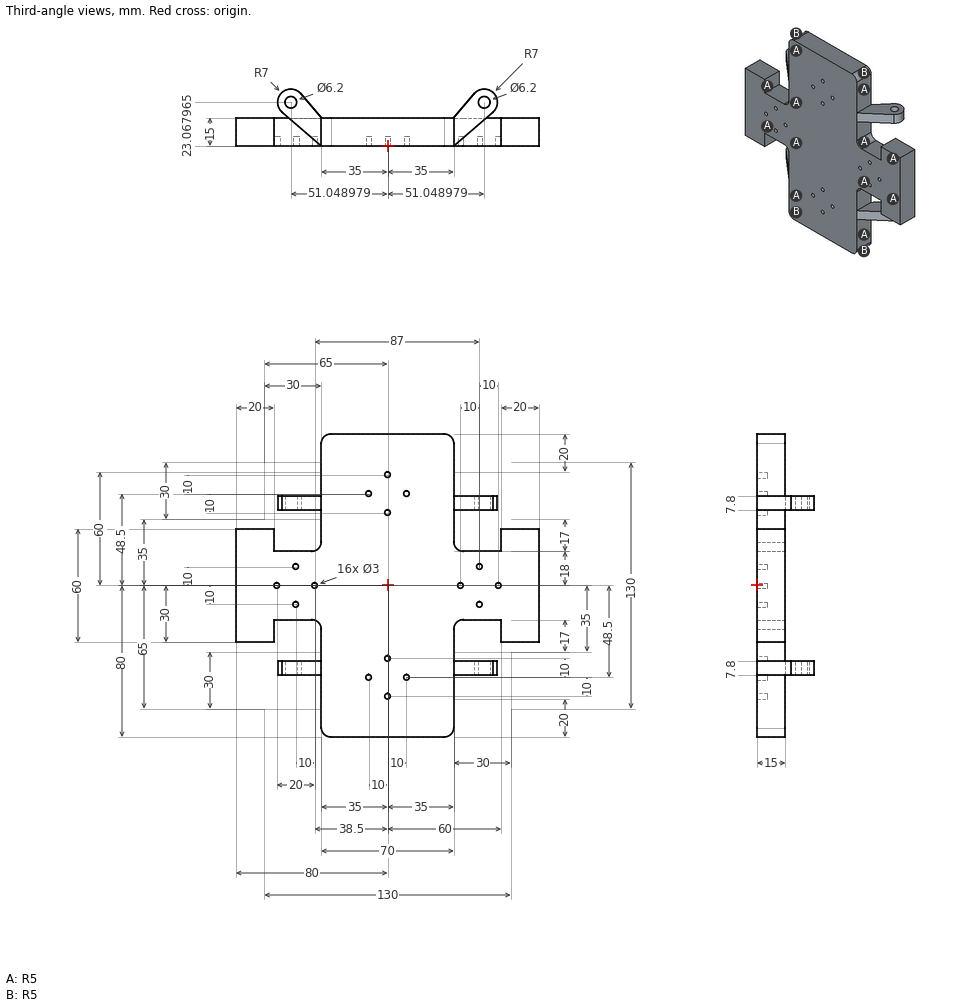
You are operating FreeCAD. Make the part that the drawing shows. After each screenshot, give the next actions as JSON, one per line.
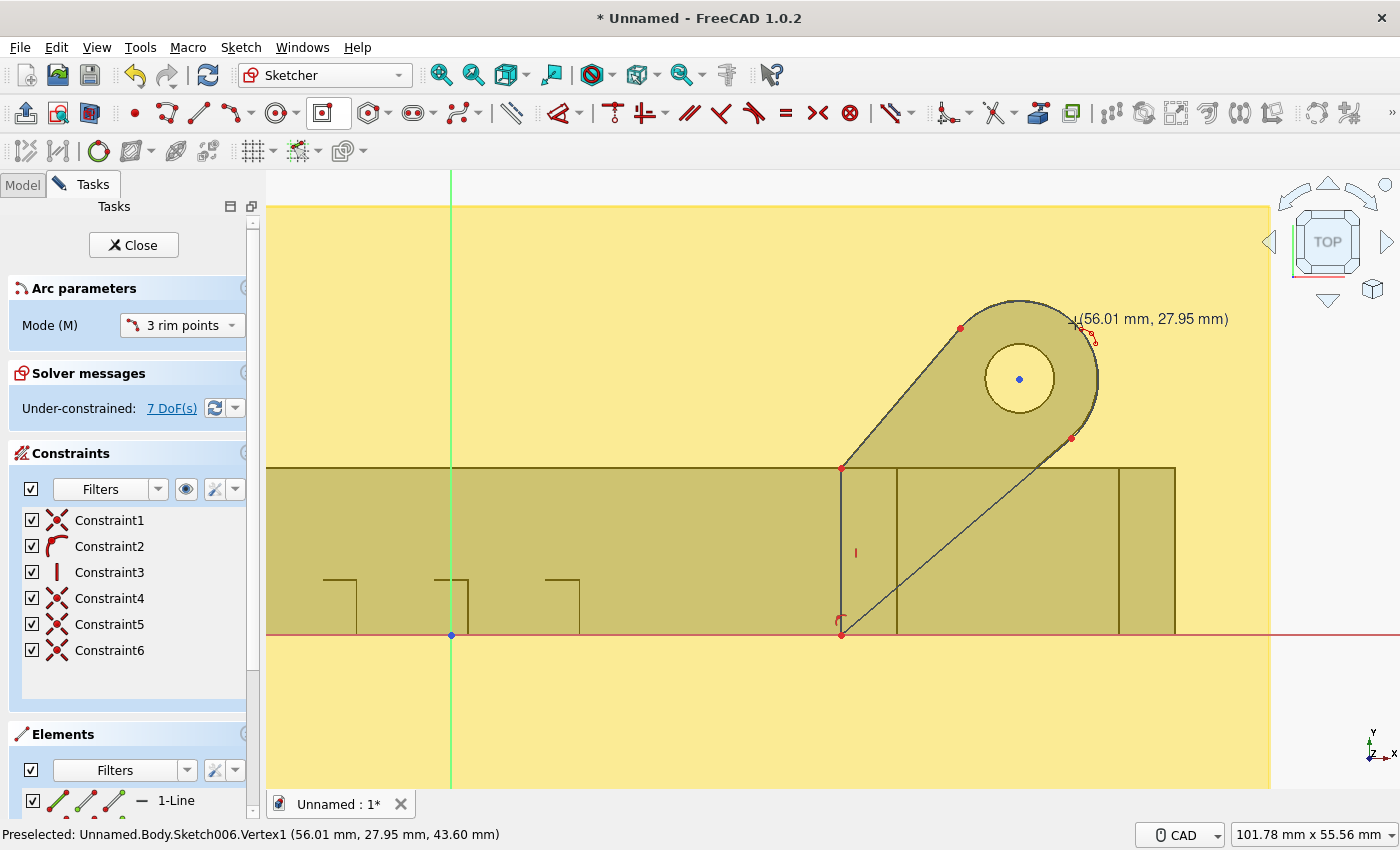
{"action": "left_click", "coordinate": [276, 114]}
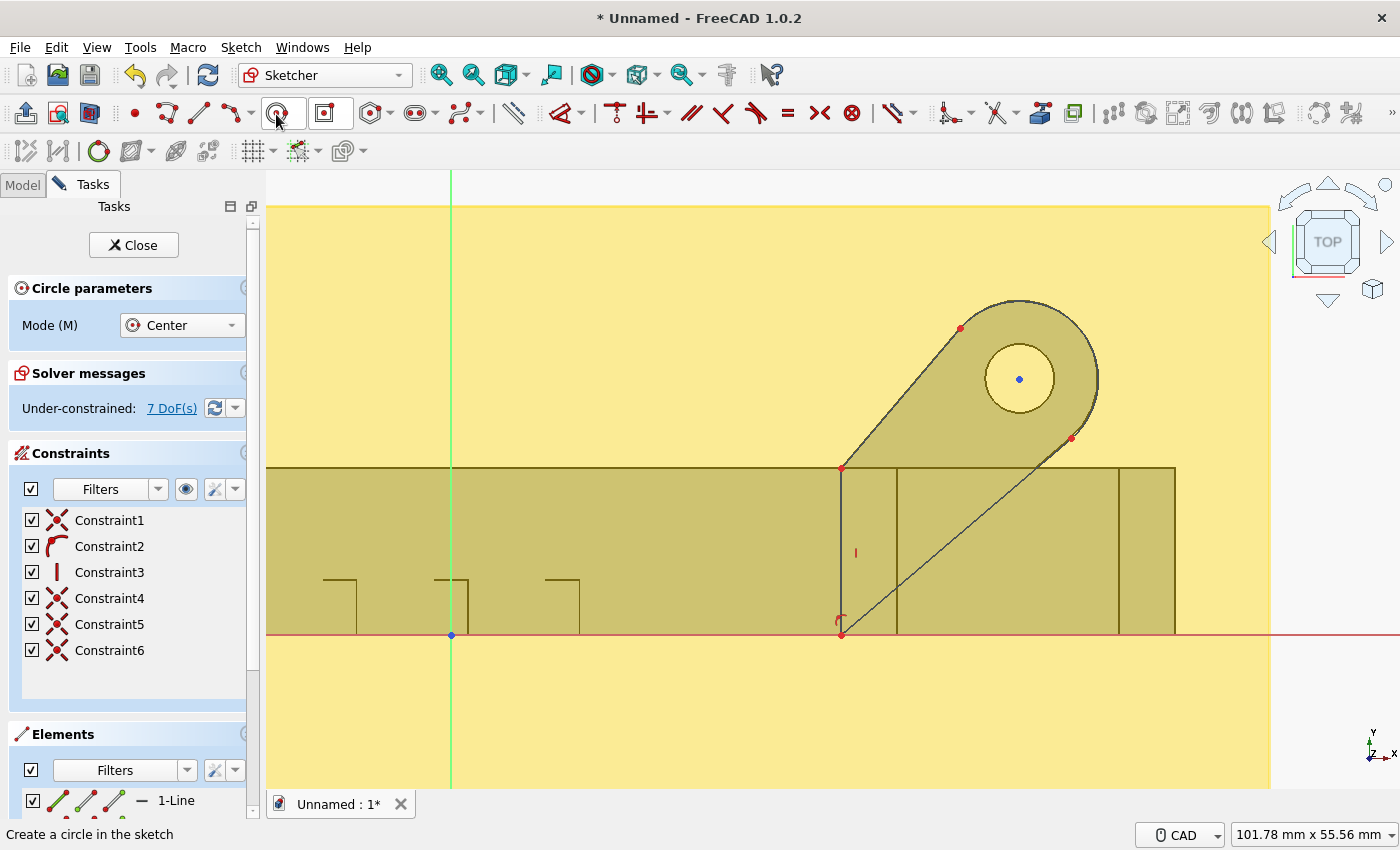
{"action": "left_click", "coordinate": [1020, 378]}
{"action": "mouse_move", "coordinate": [1044, 354]}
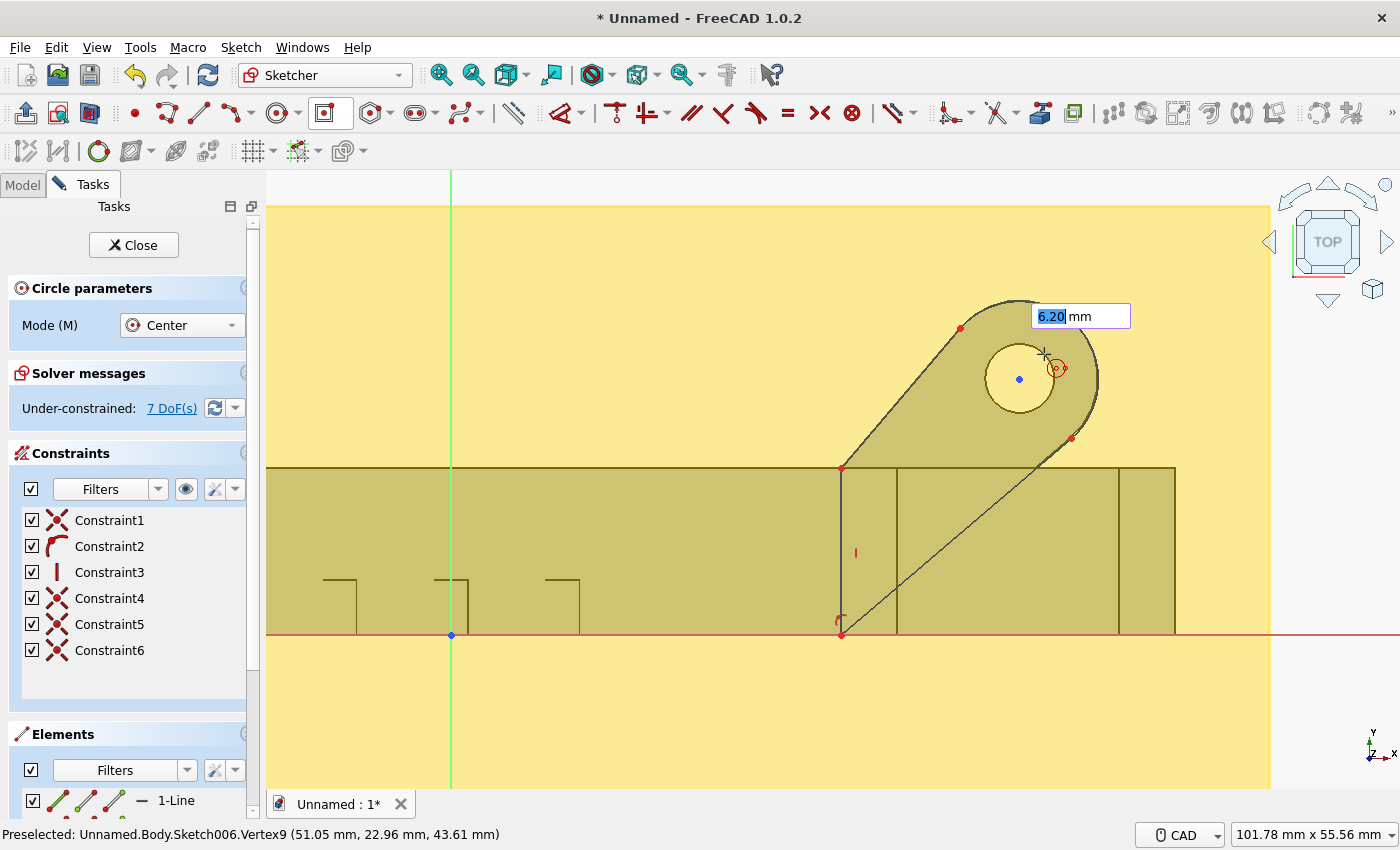
{"action": "type", "text": "6.2"}
{"action": "key", "text": "Return"}
{"action": "key", "text": "Escape"}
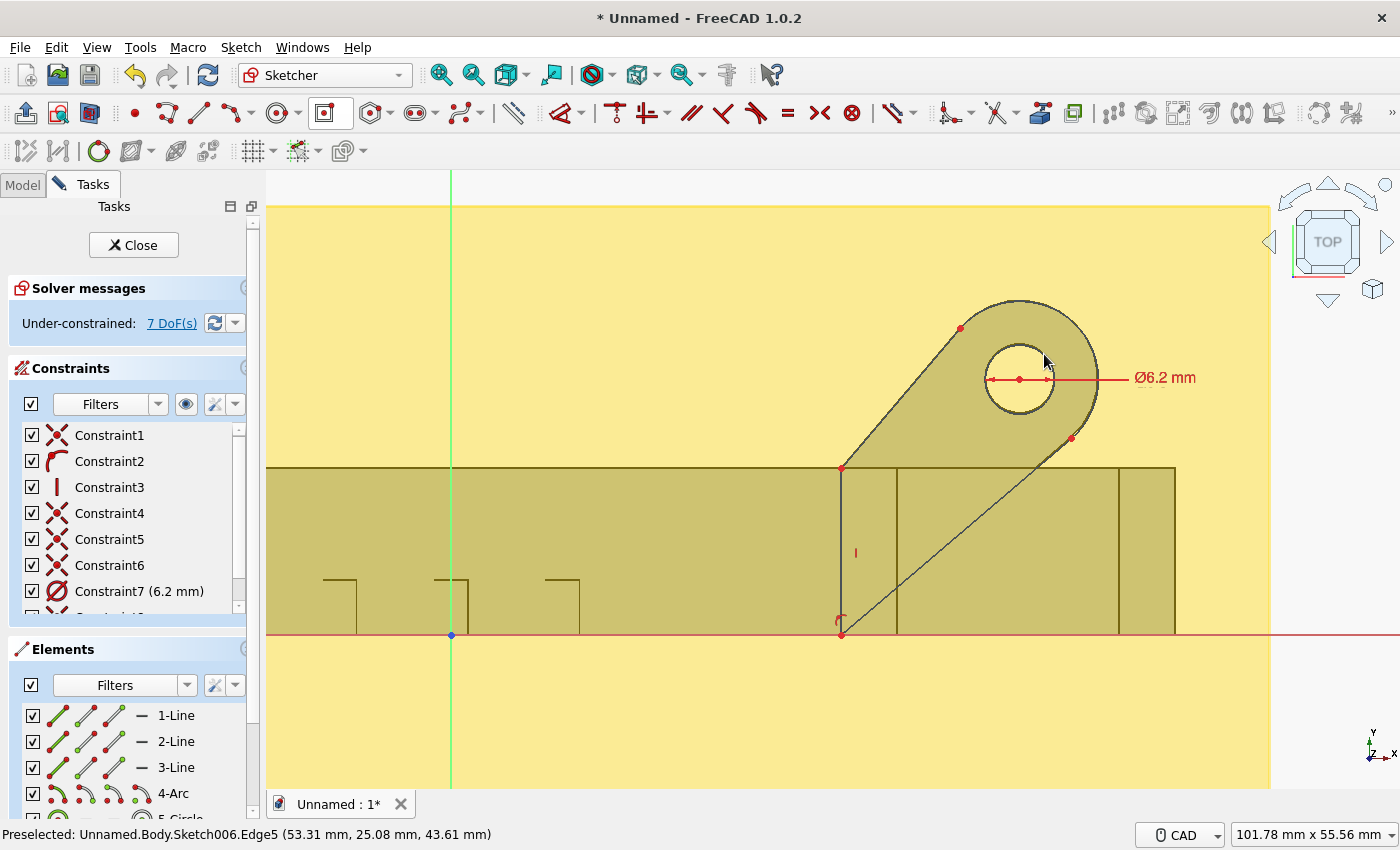
{"action": "left_click", "coordinate": [924, 371]}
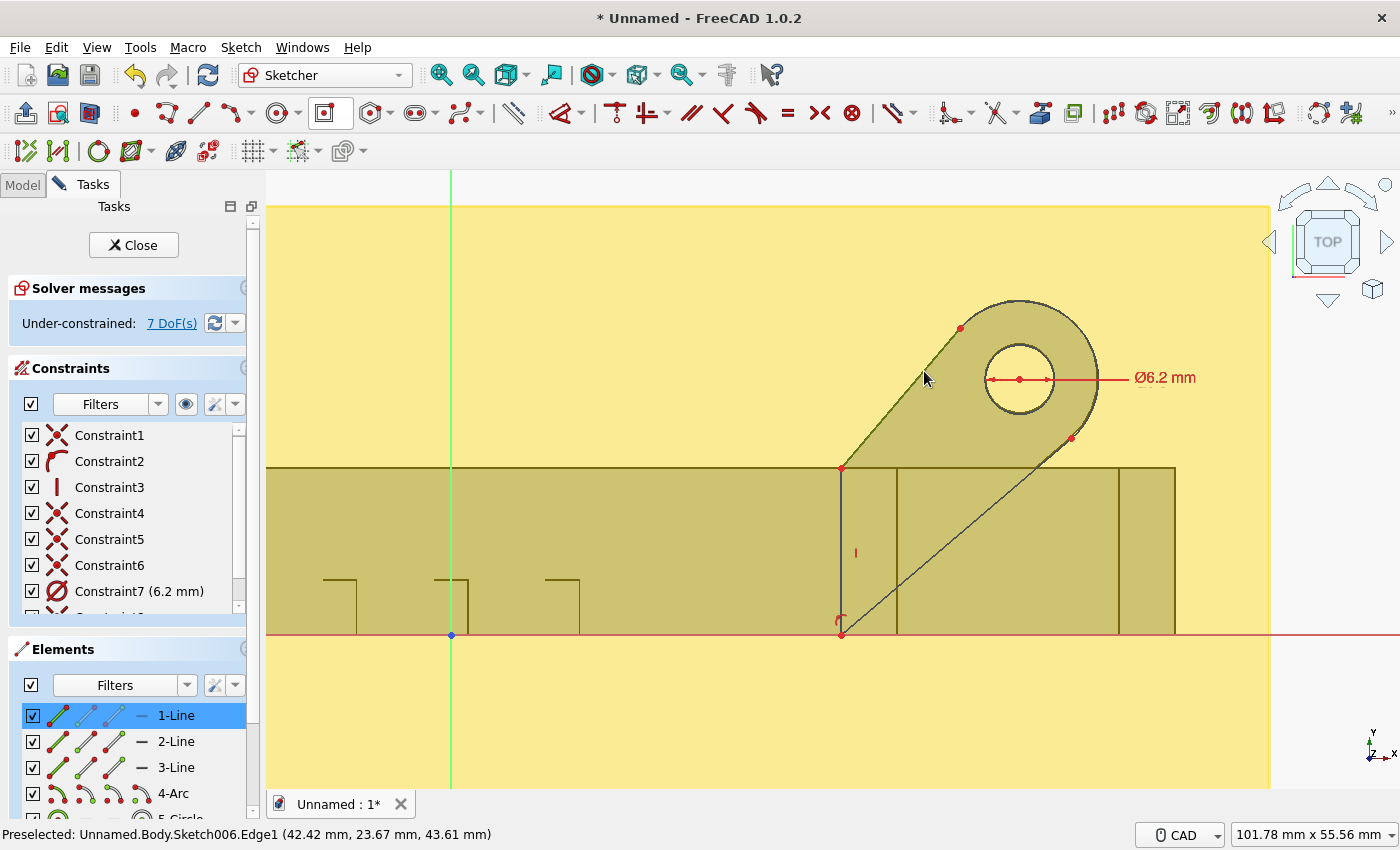
{"action": "left_click", "coordinate": [1098, 369]}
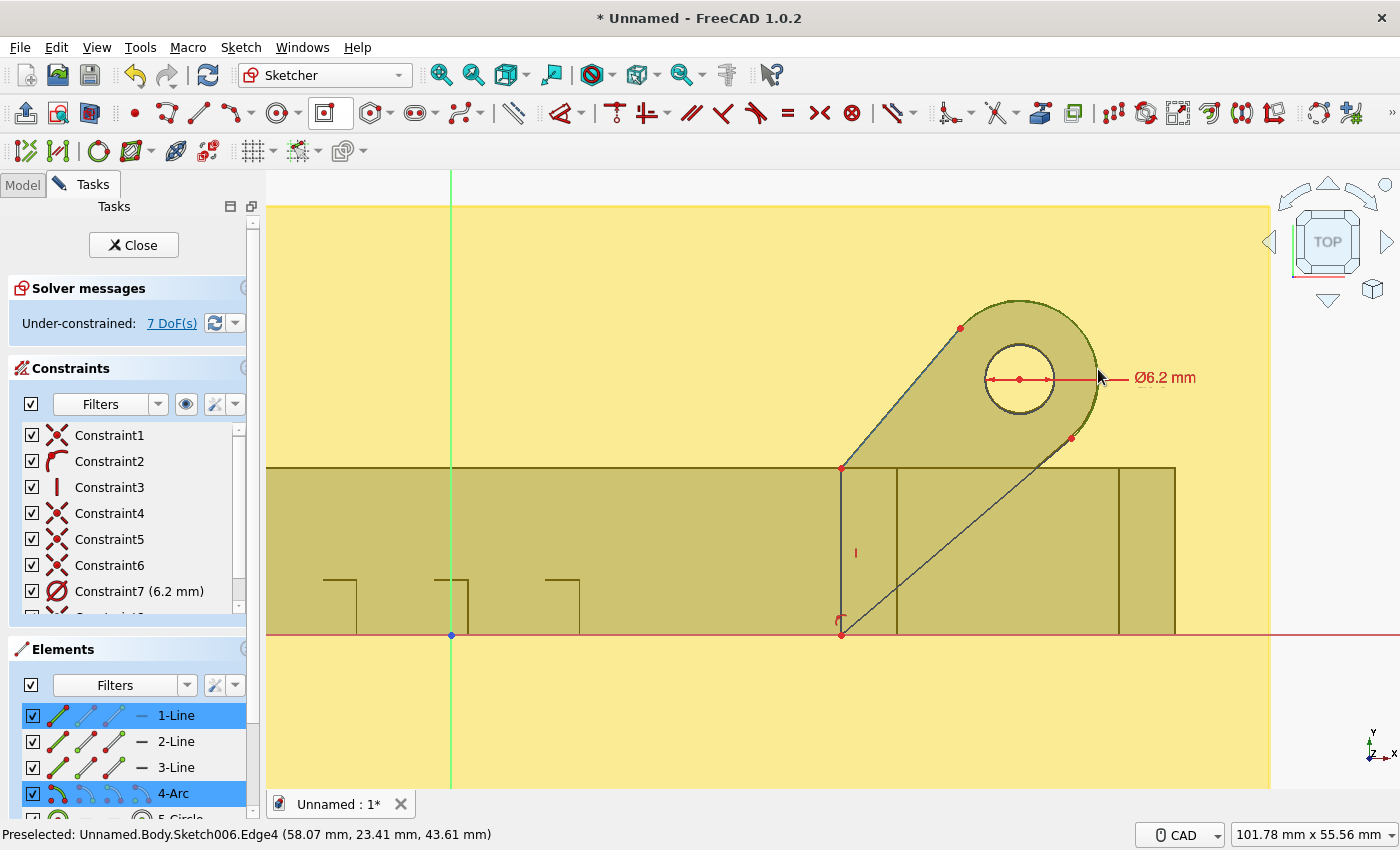
{"action": "key", "text": "t"}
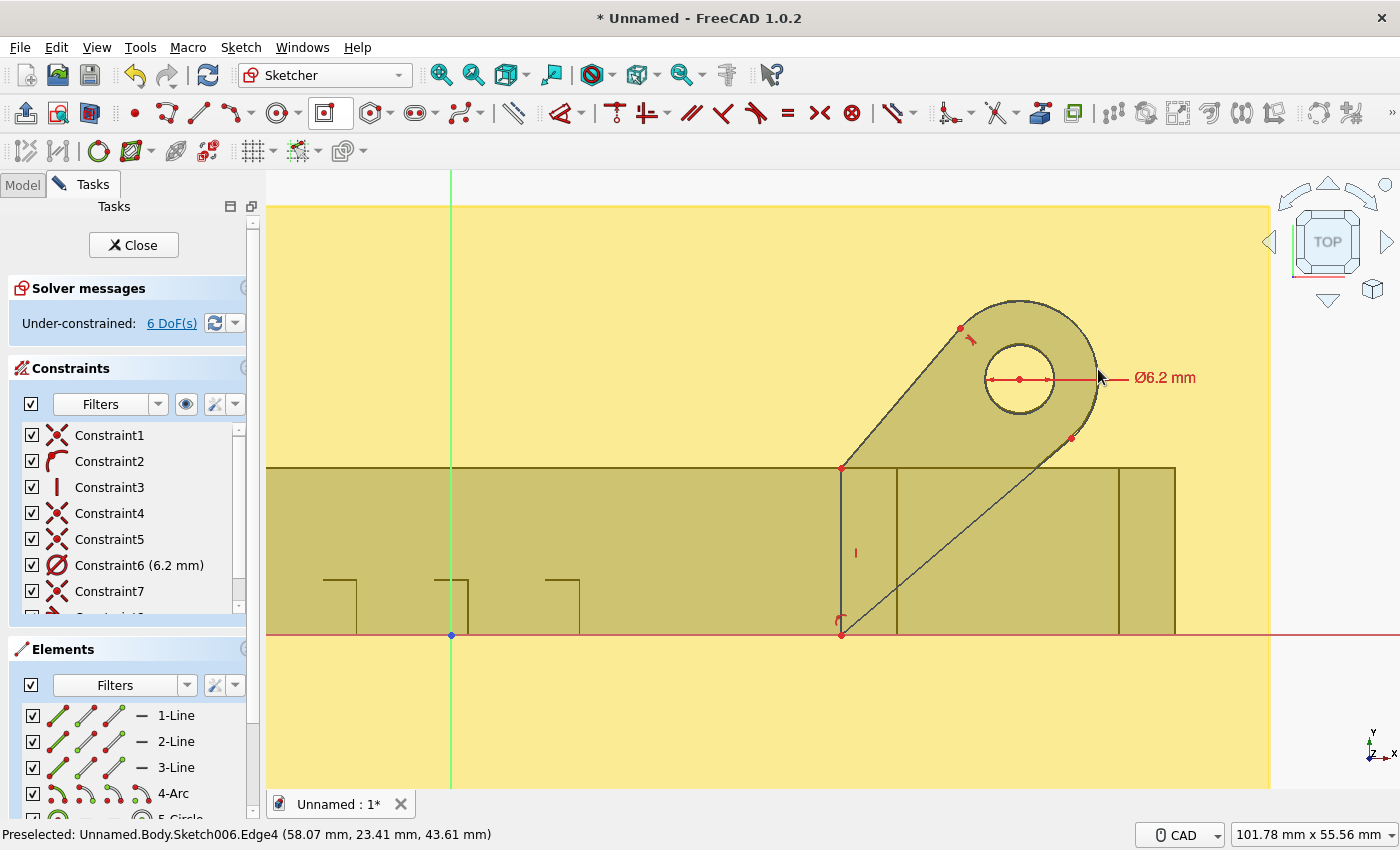
{"action": "left_click", "coordinate": [910, 577]}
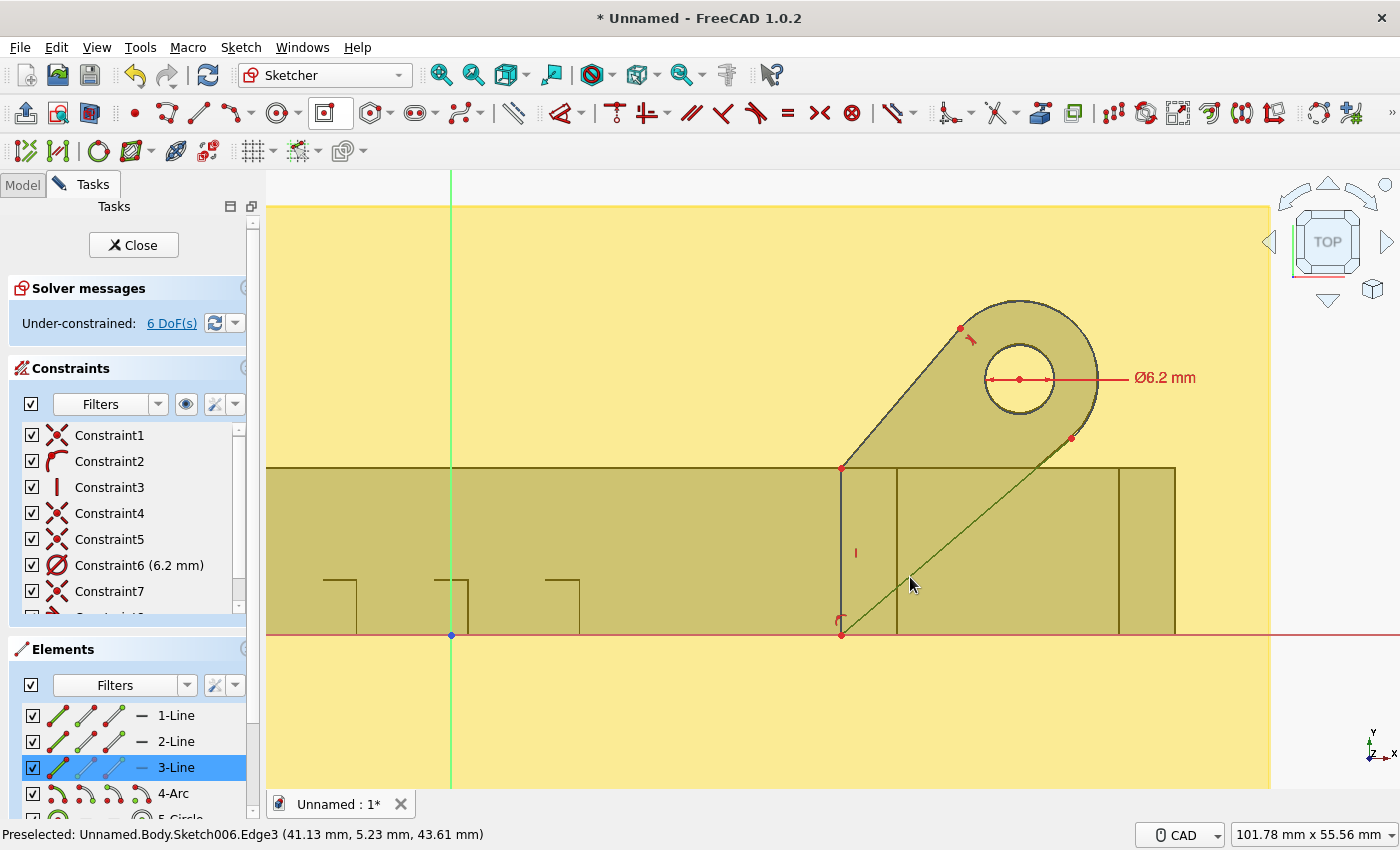
{"action": "left_click", "coordinate": [1097, 370]}